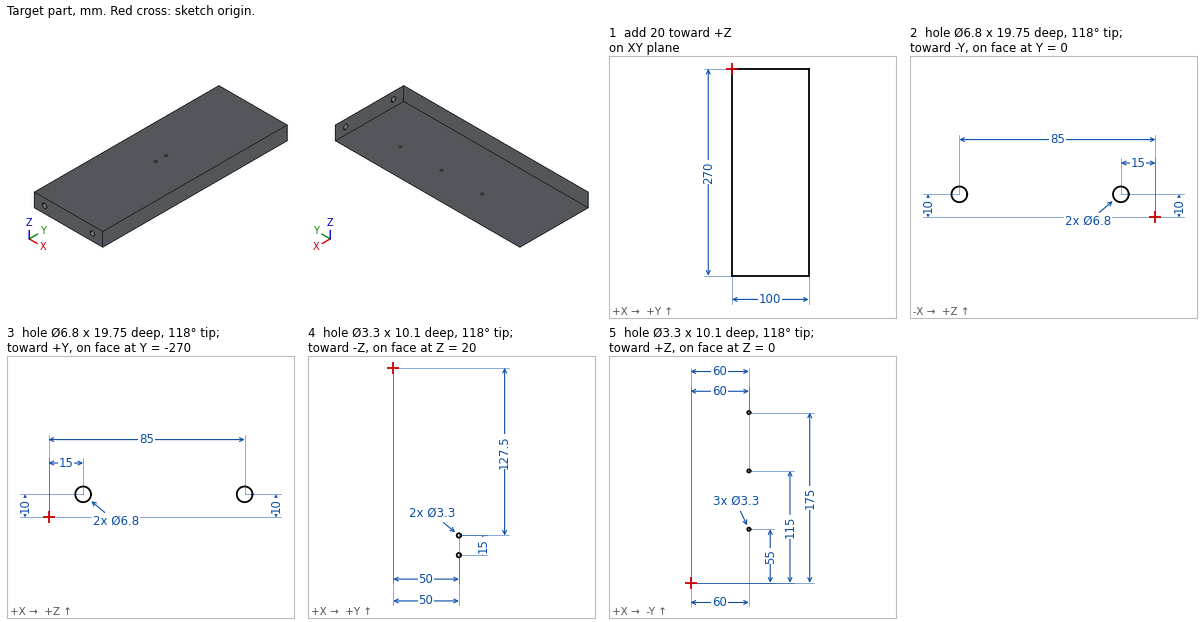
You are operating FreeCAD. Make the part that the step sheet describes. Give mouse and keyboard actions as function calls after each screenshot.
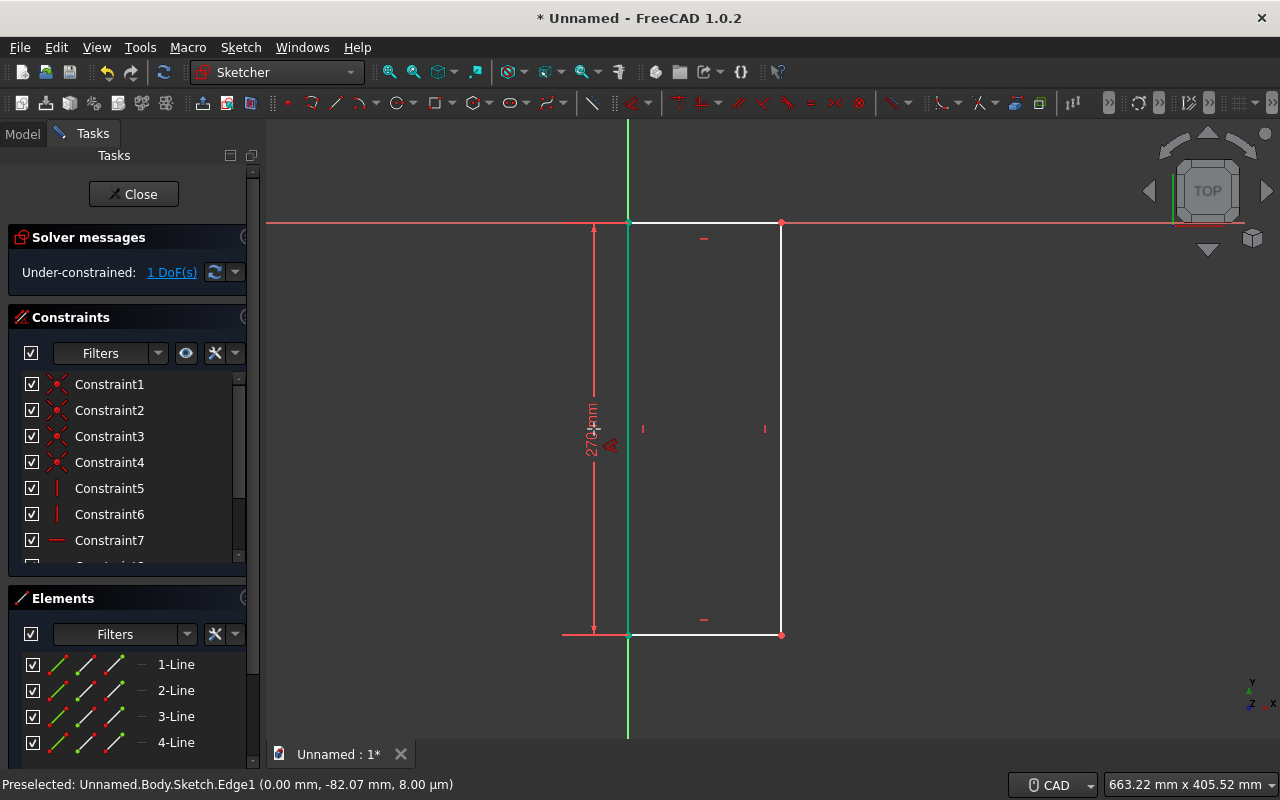
click(674, 635)
click(705, 669)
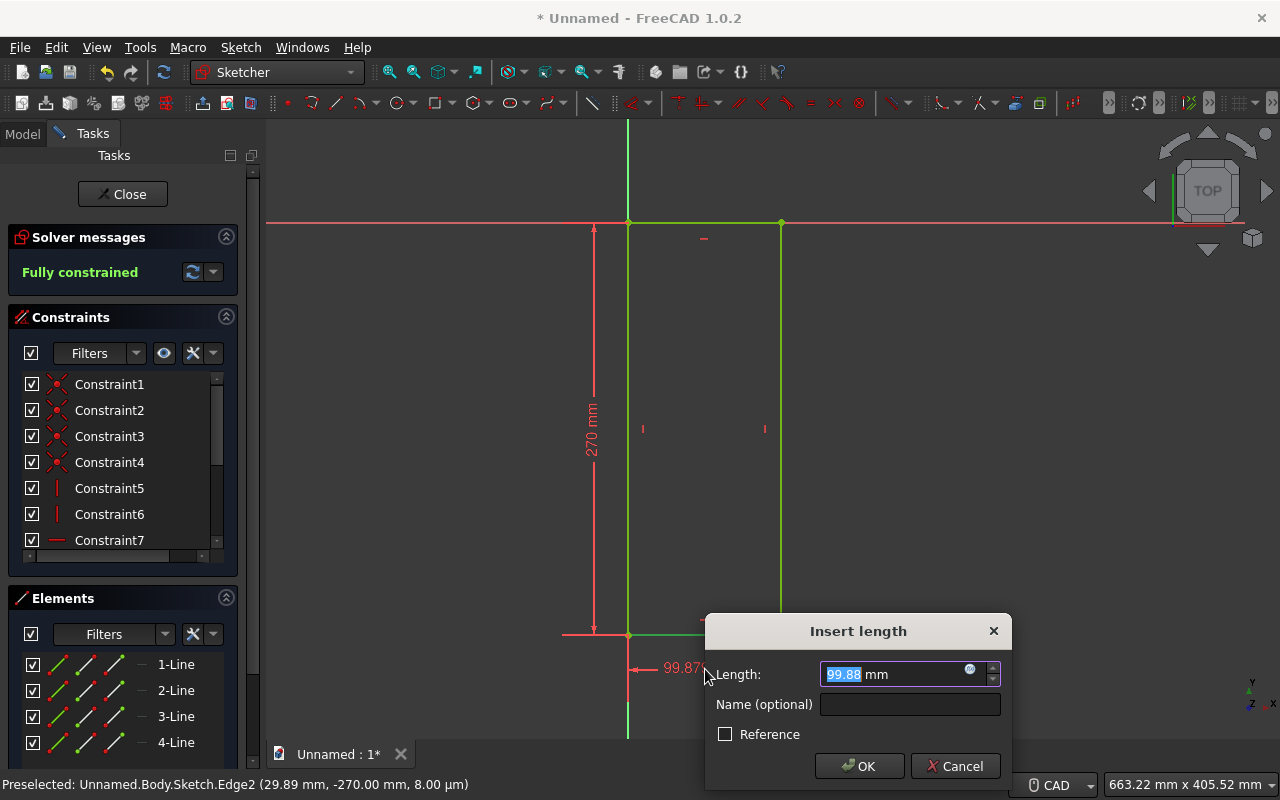
text(100)
key(Return)
key(Escape)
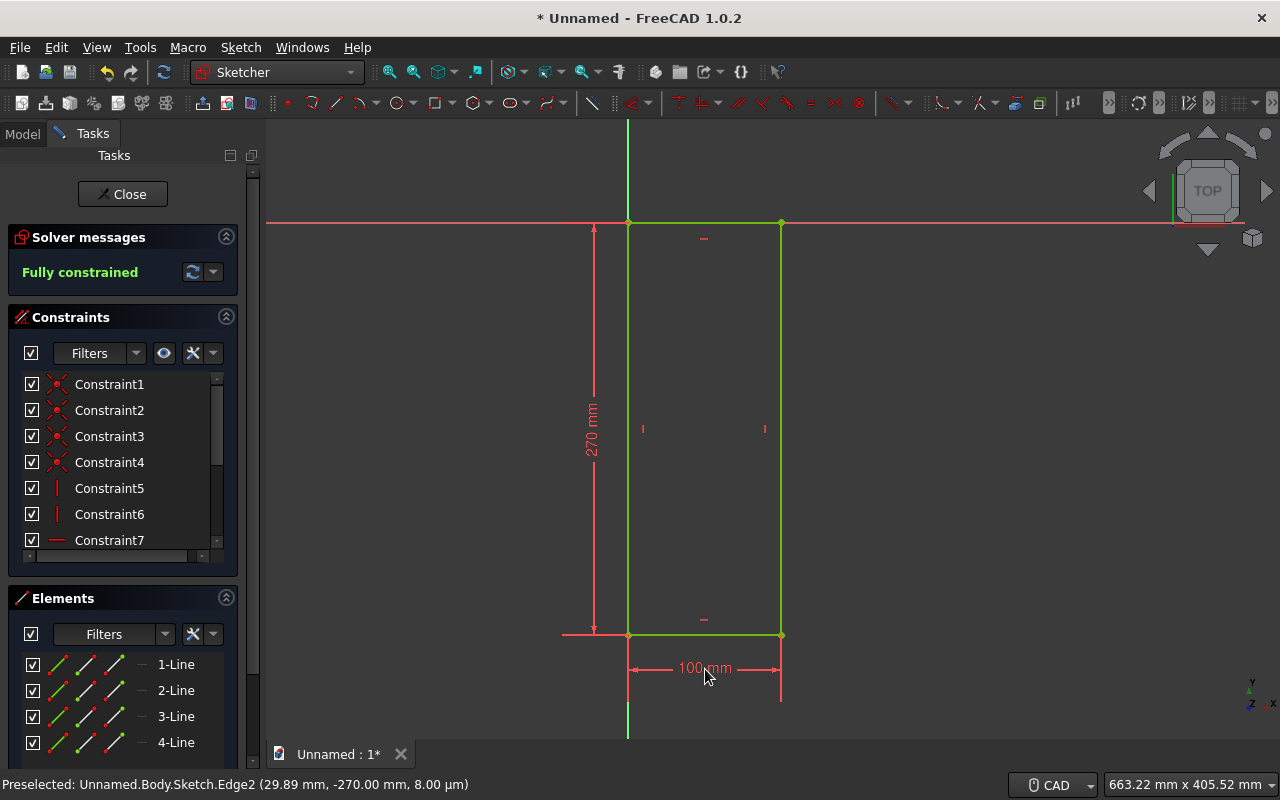
click(123, 194)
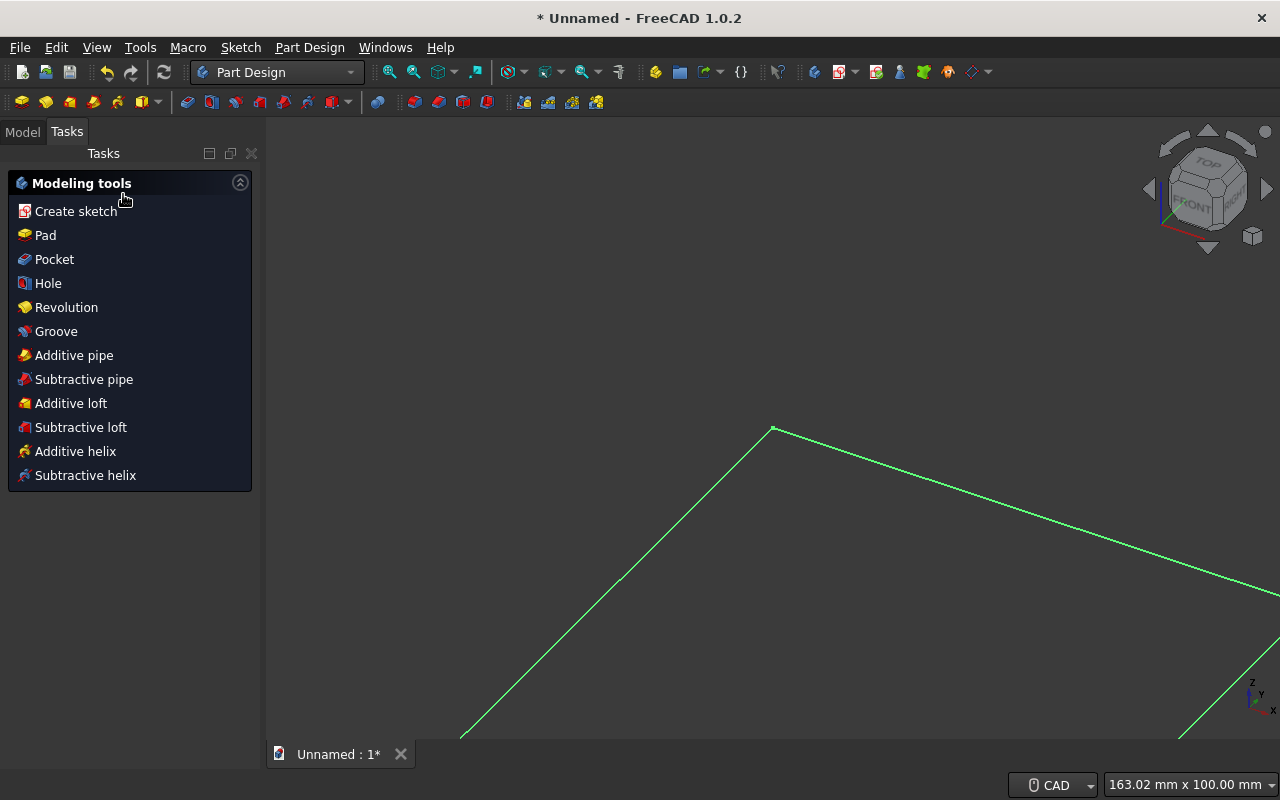
click(22, 102)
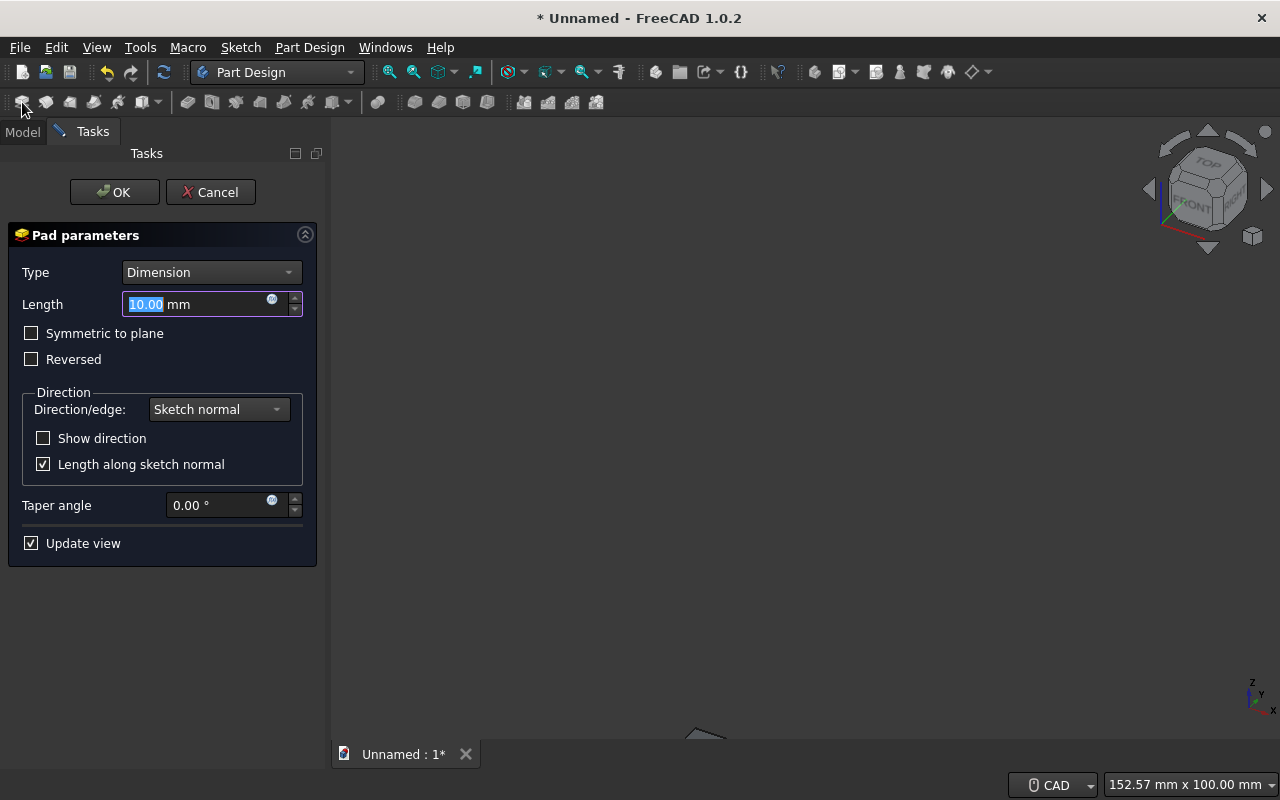
text(20)
key(Tab)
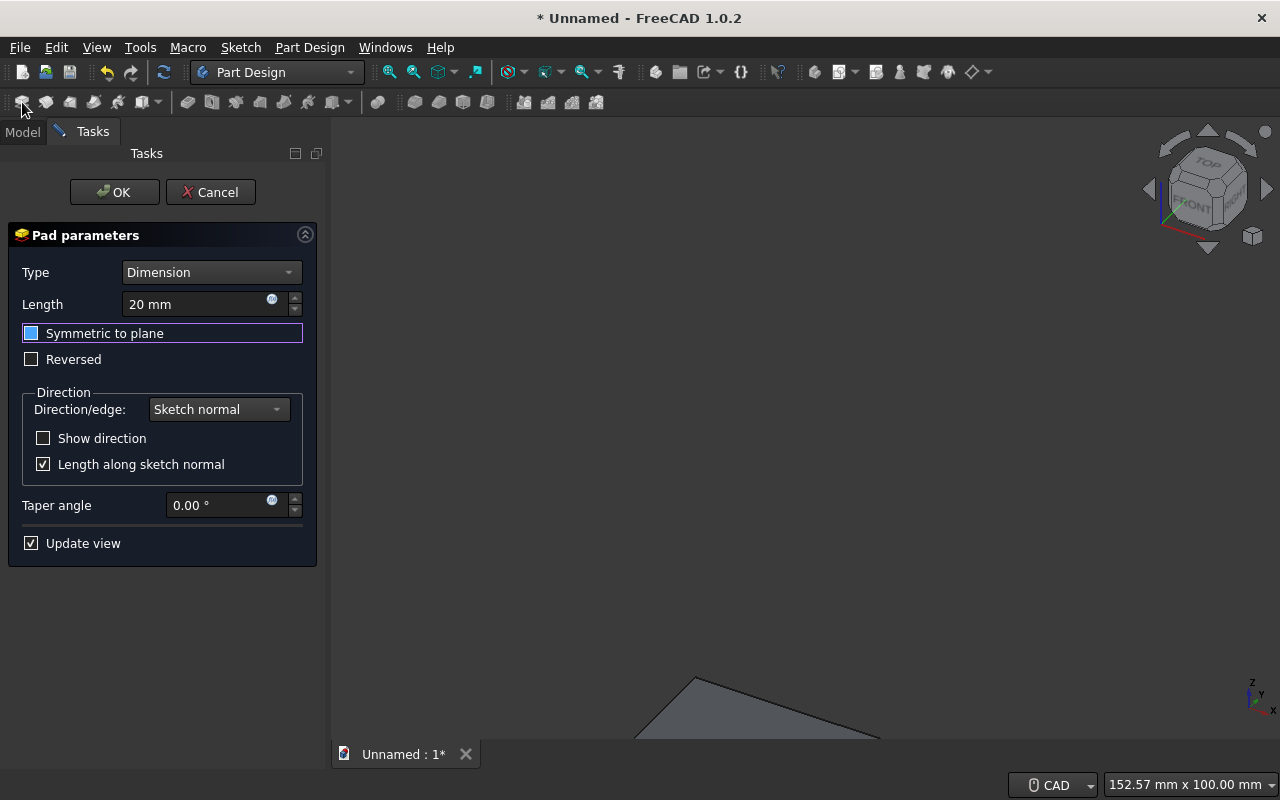
click(115, 192)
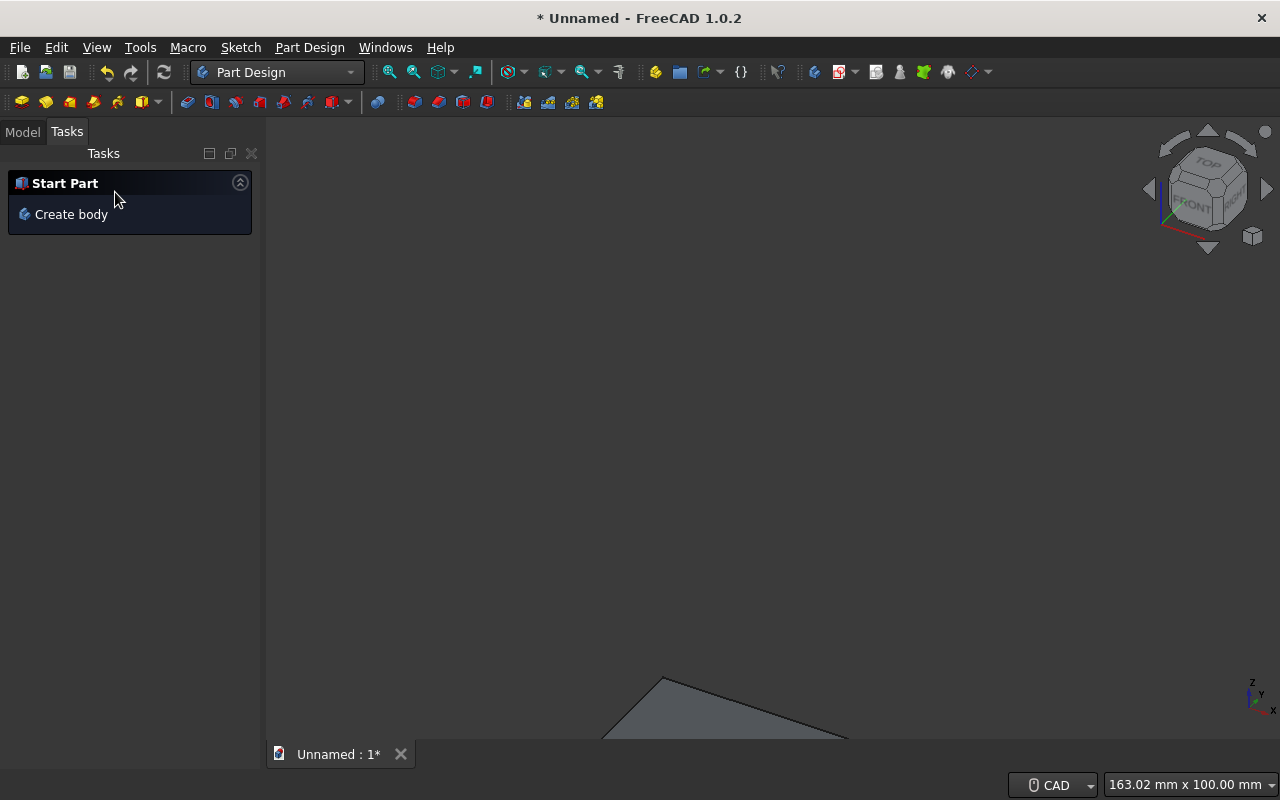
click(390, 72)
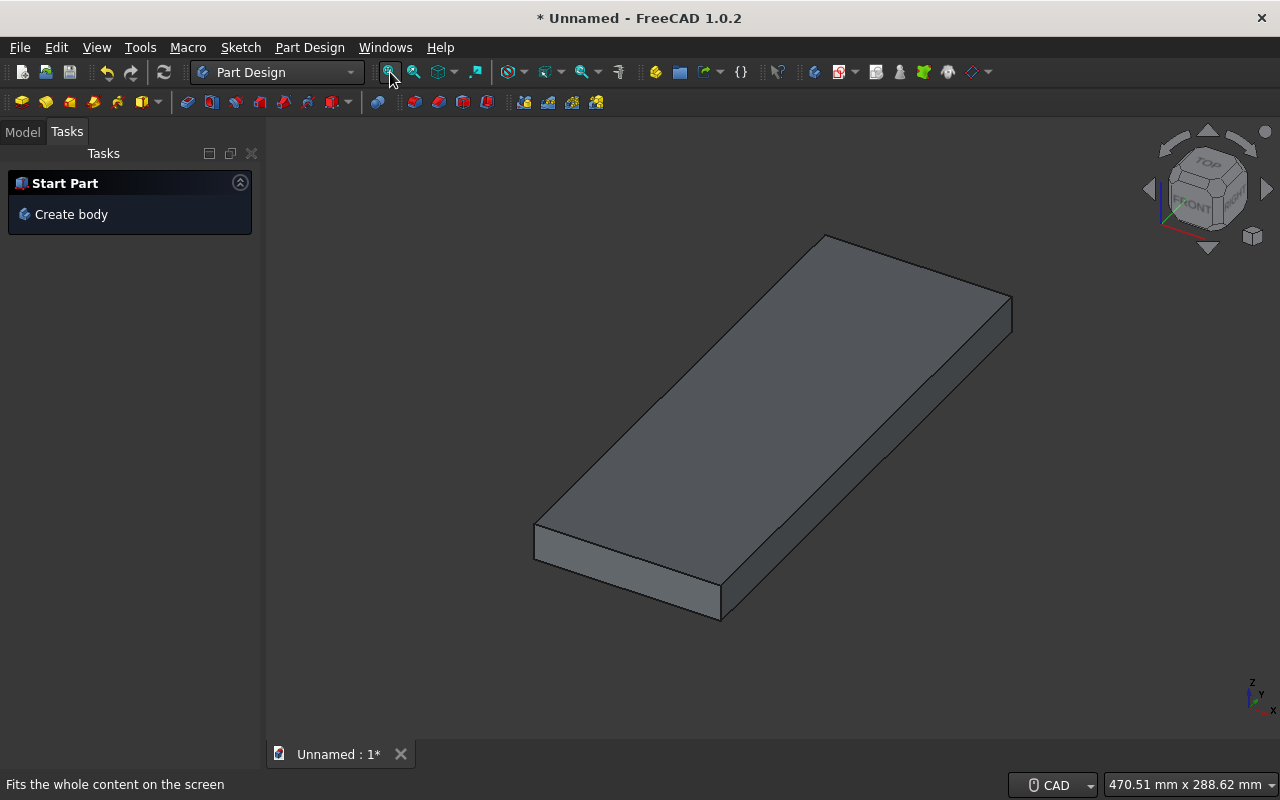
key(4)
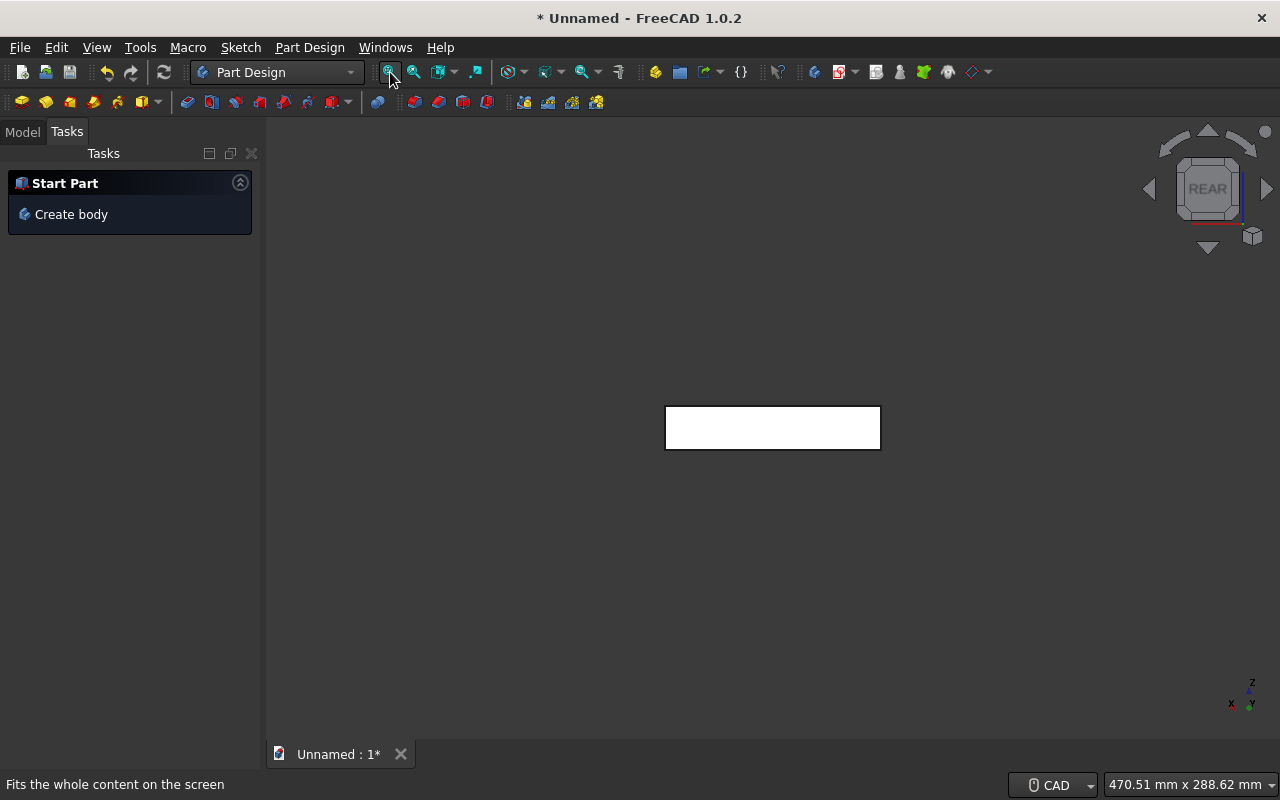
key(v)
key(f)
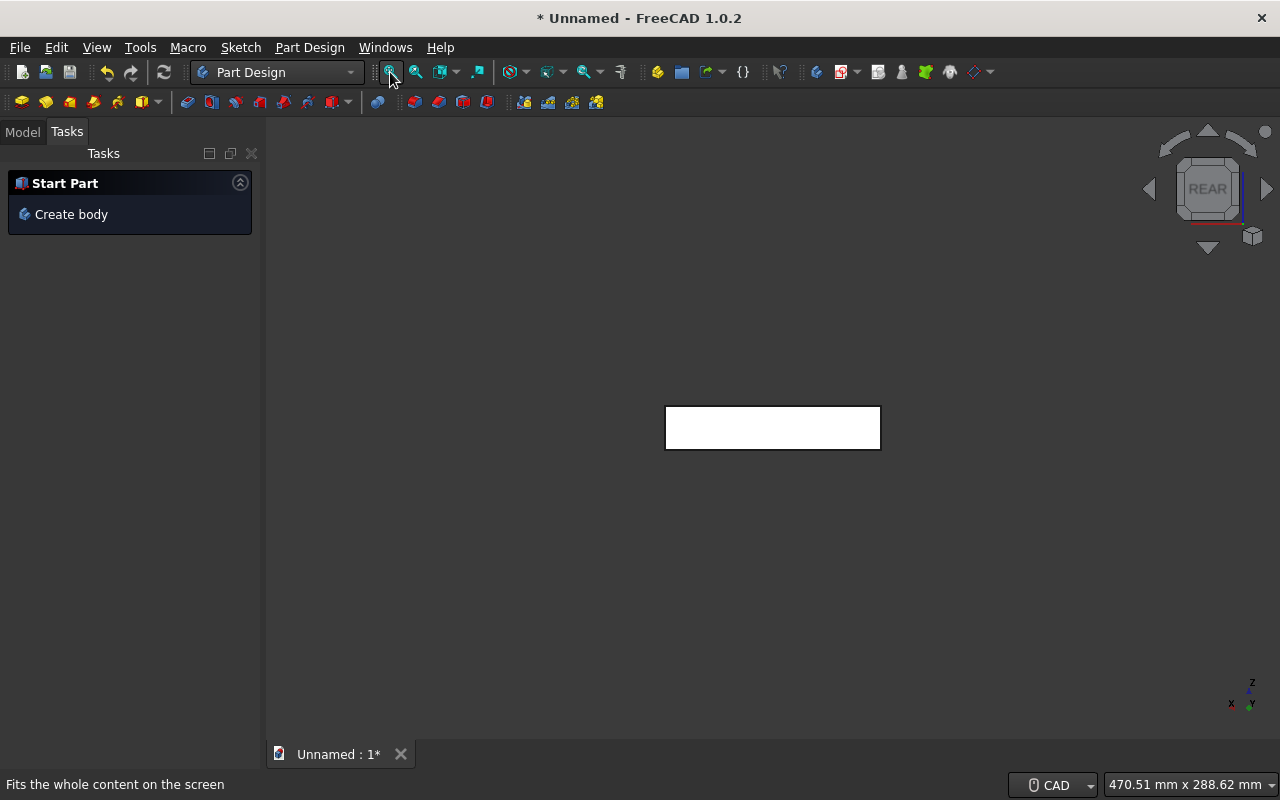
click(711, 427)